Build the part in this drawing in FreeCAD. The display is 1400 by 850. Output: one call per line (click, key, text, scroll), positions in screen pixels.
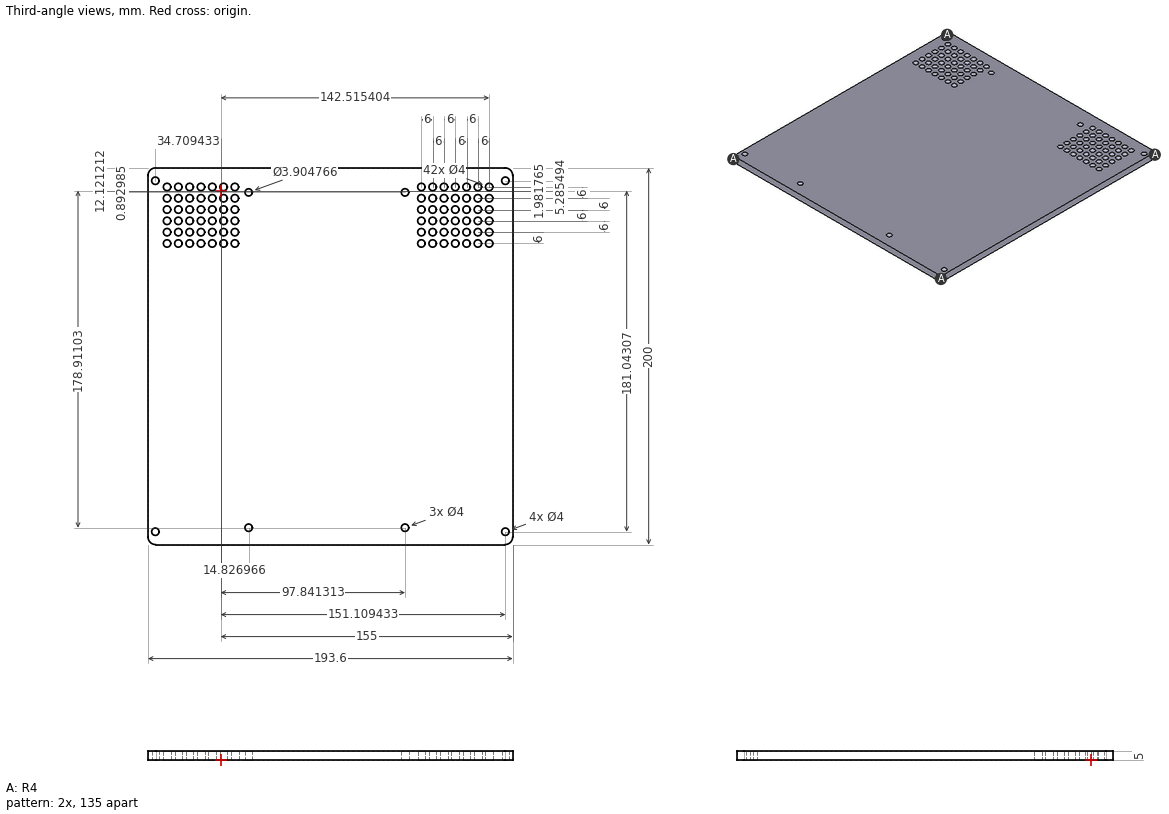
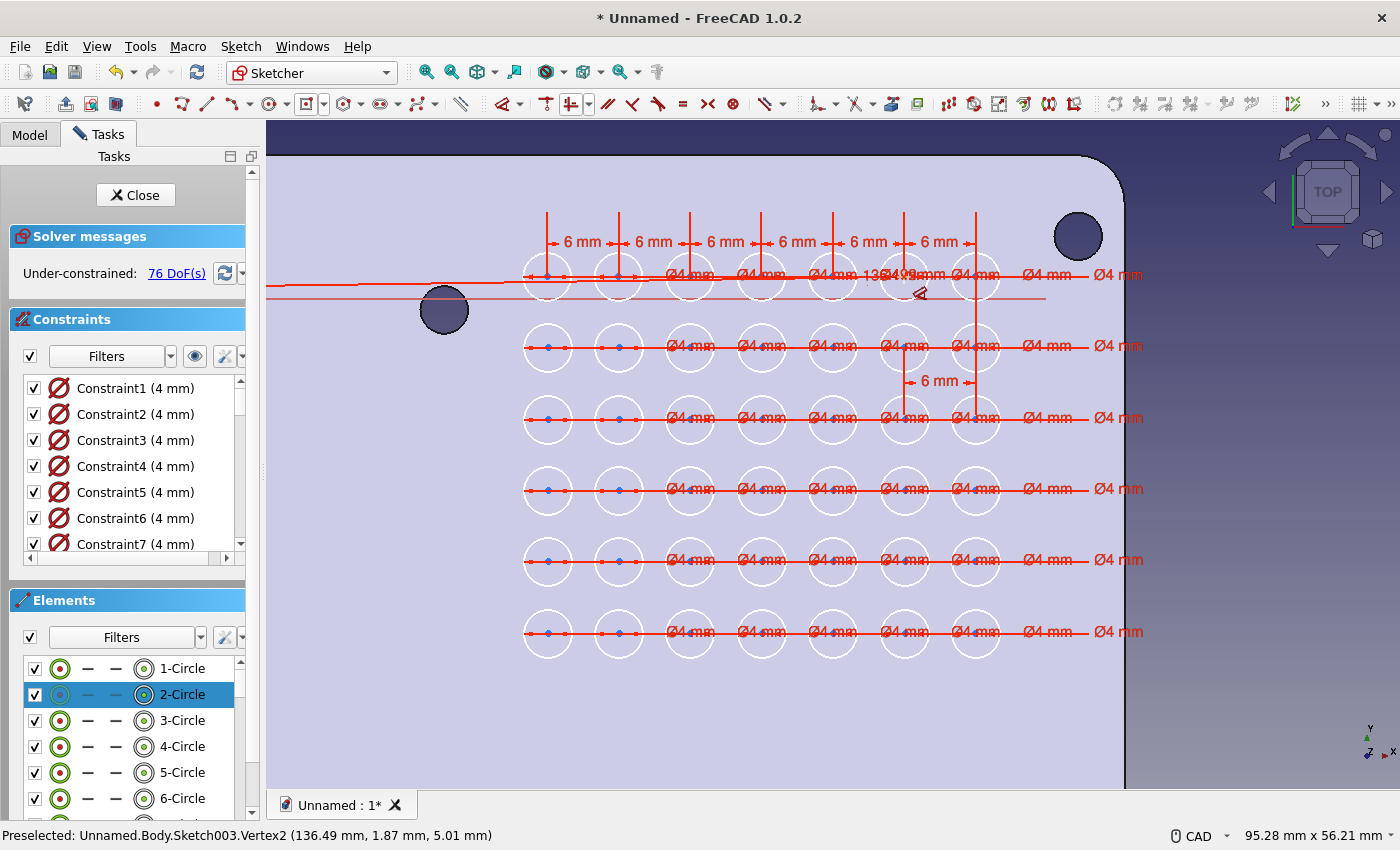
click(904, 348)
click(938, 313)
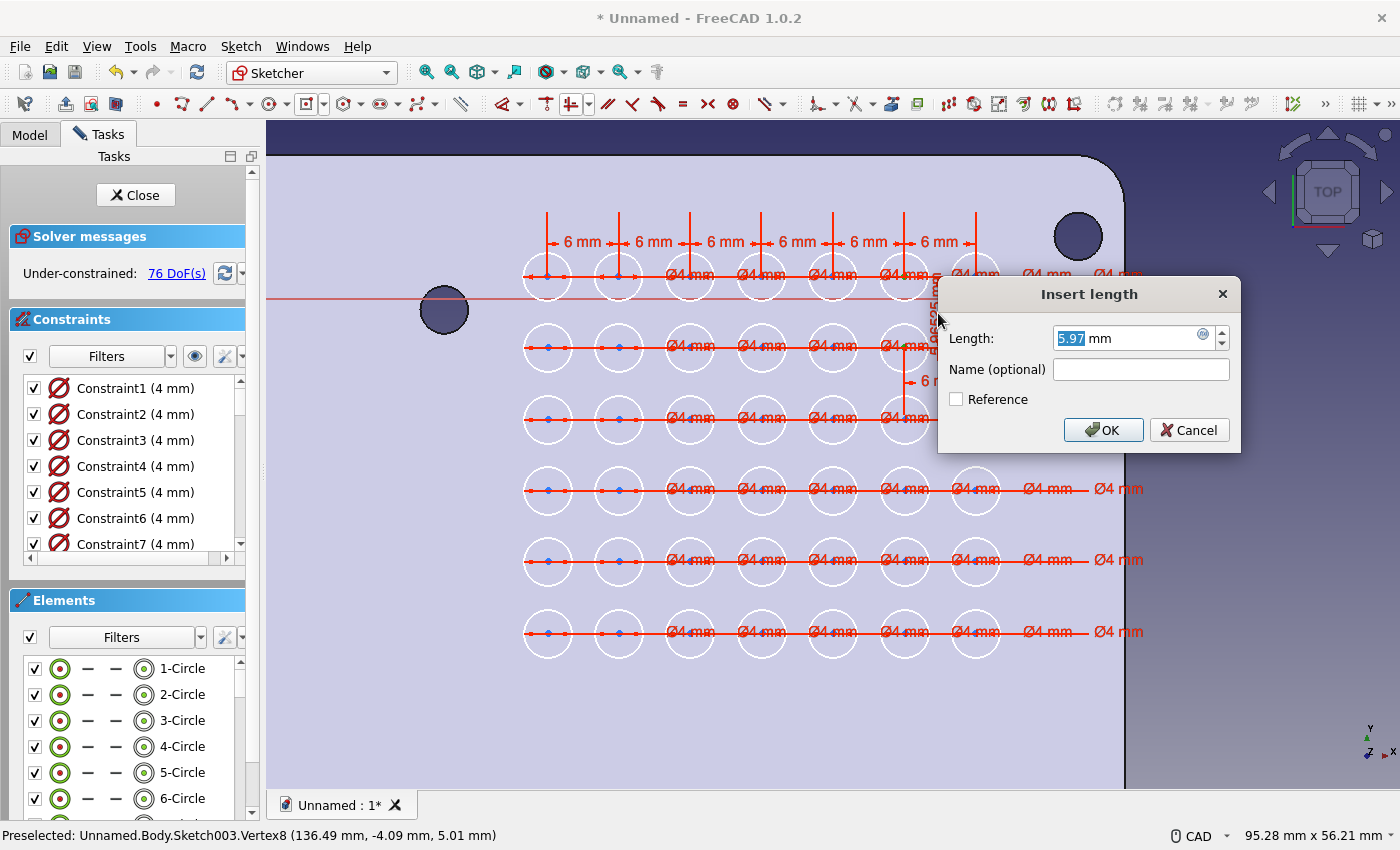
text(6)
key(Return)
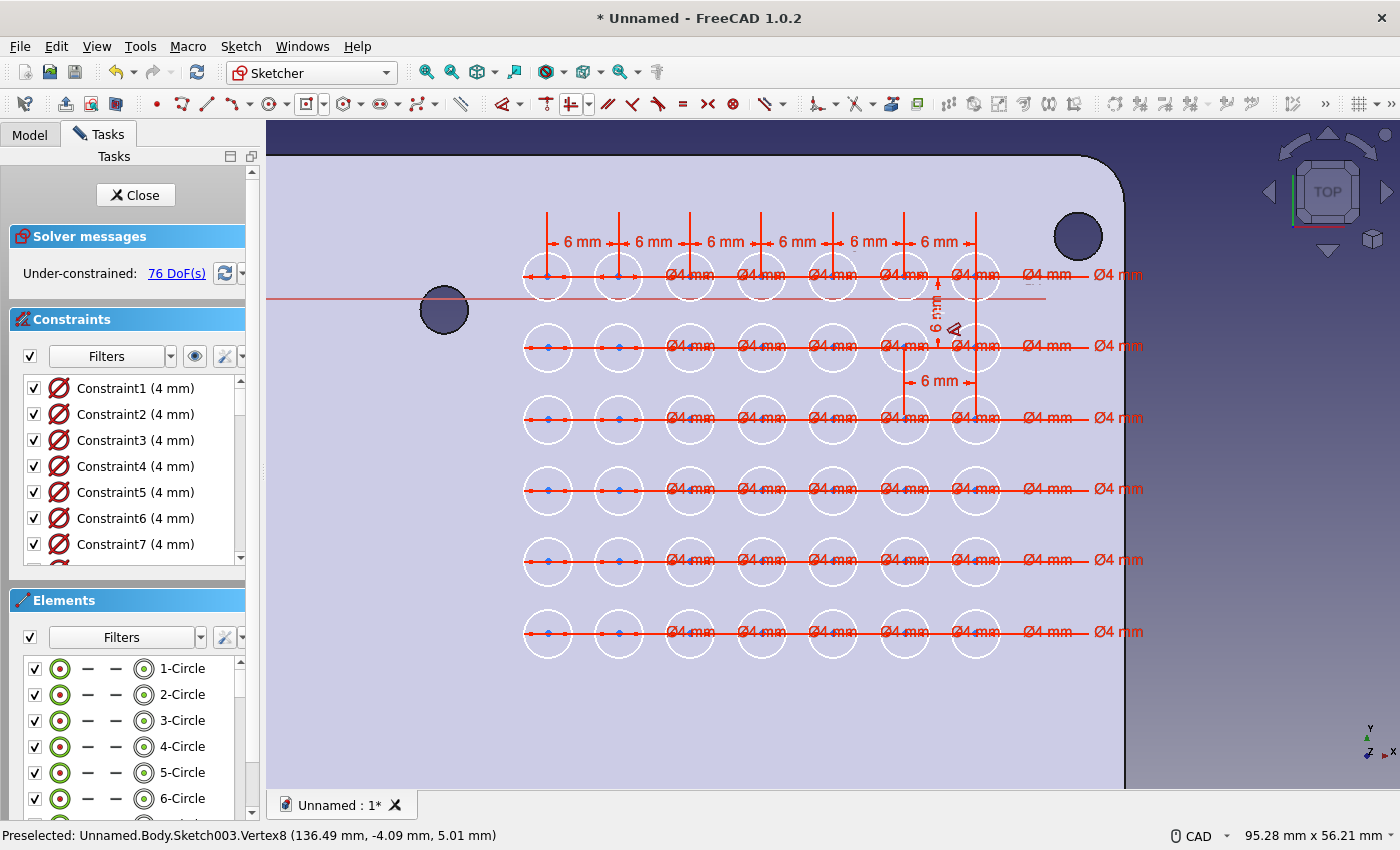
click(976, 277)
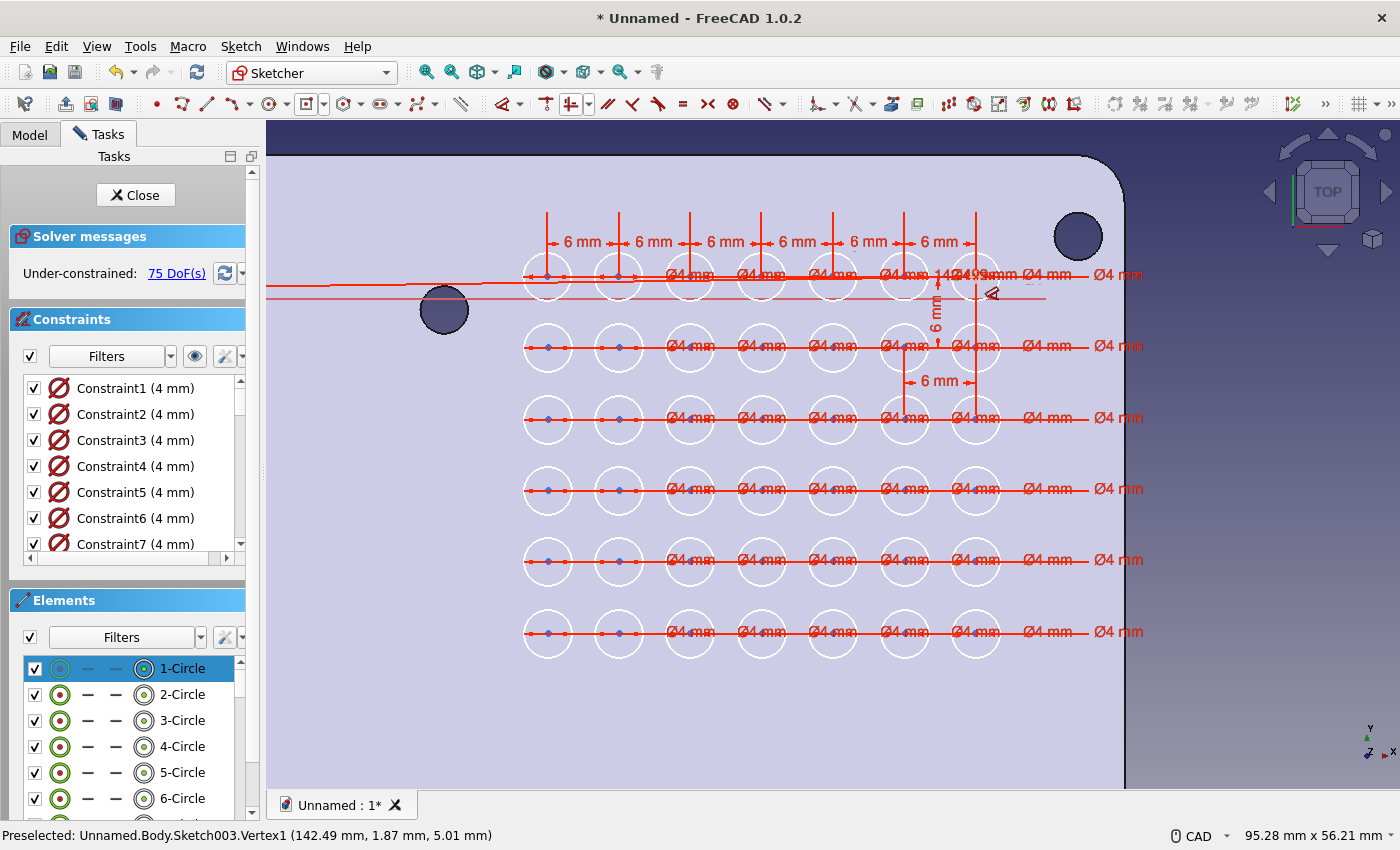
click(904, 348)
click(1010, 313)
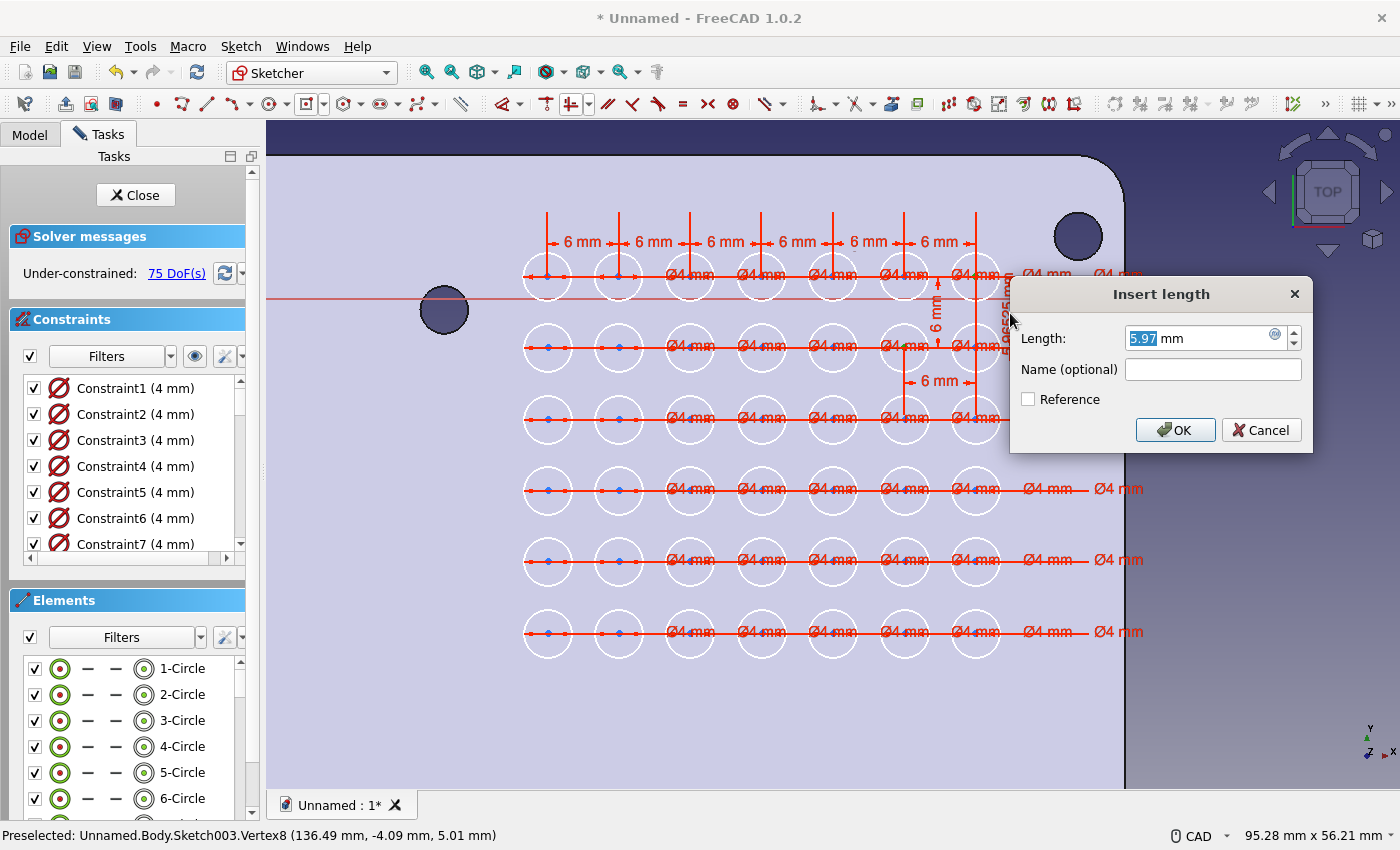
text(6)
key(Return)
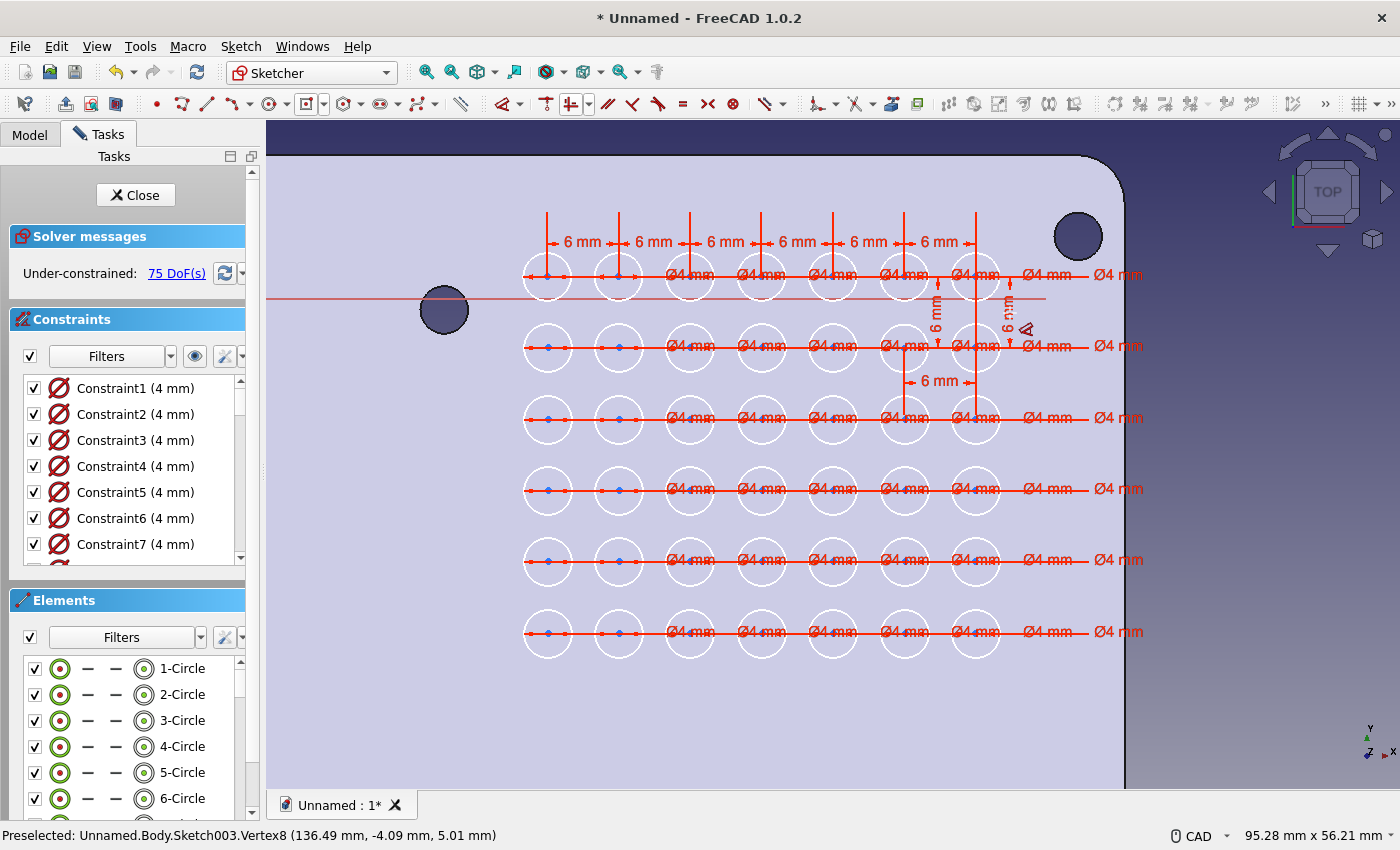
click(833, 277)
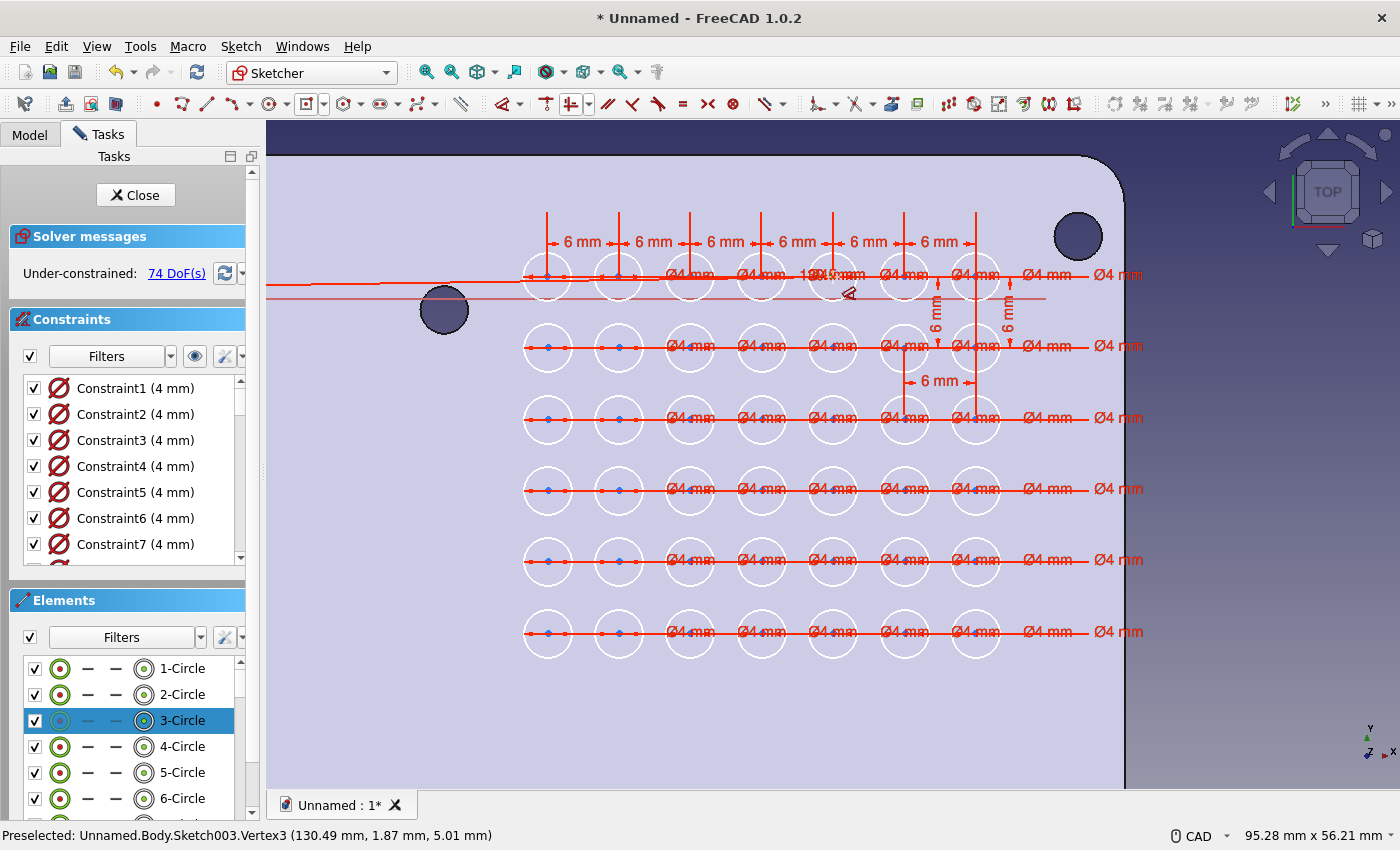
click(904, 348)
click(799, 313)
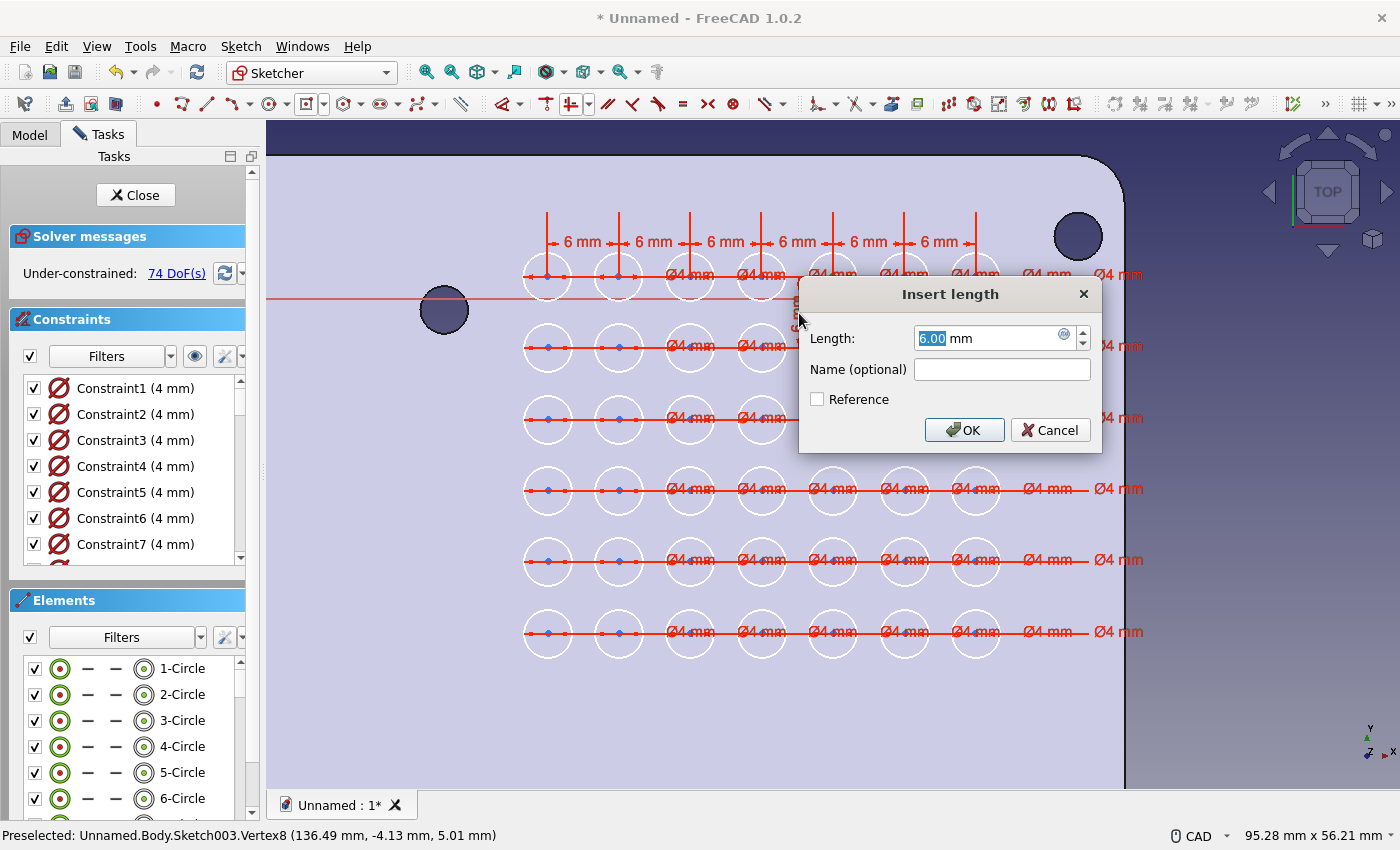
text(6)
key(Return)